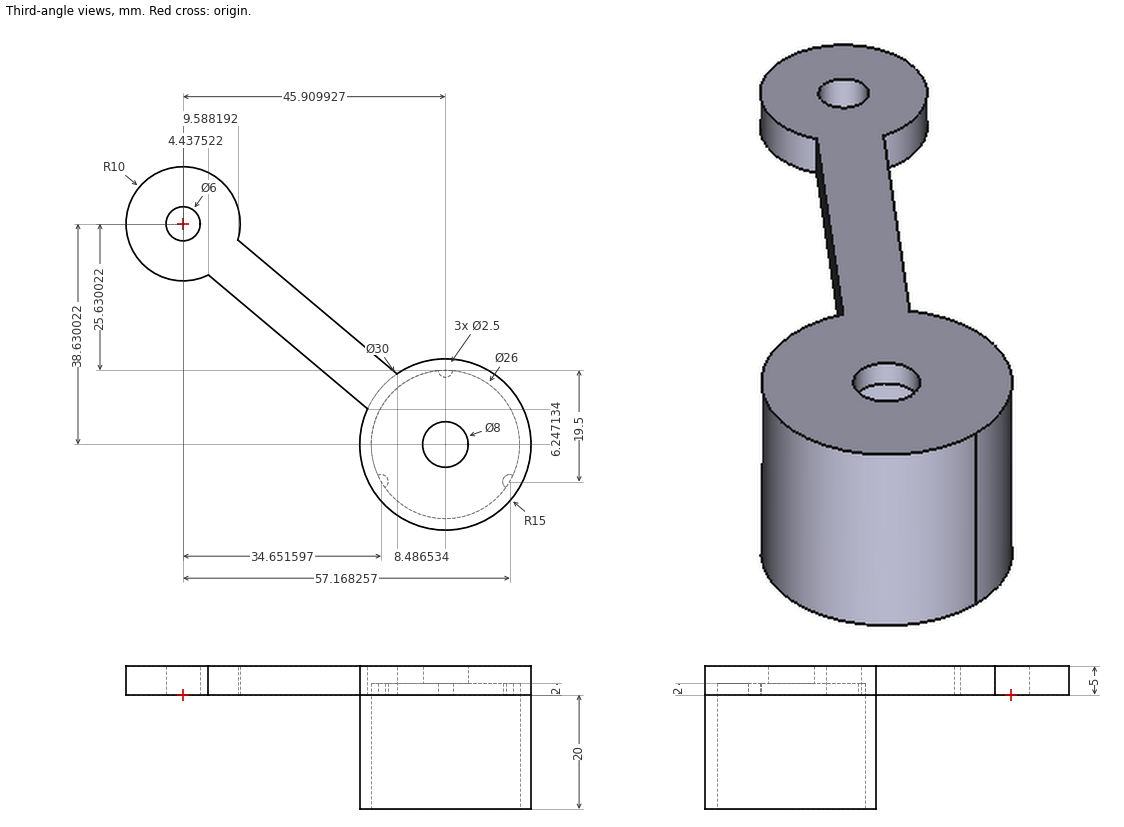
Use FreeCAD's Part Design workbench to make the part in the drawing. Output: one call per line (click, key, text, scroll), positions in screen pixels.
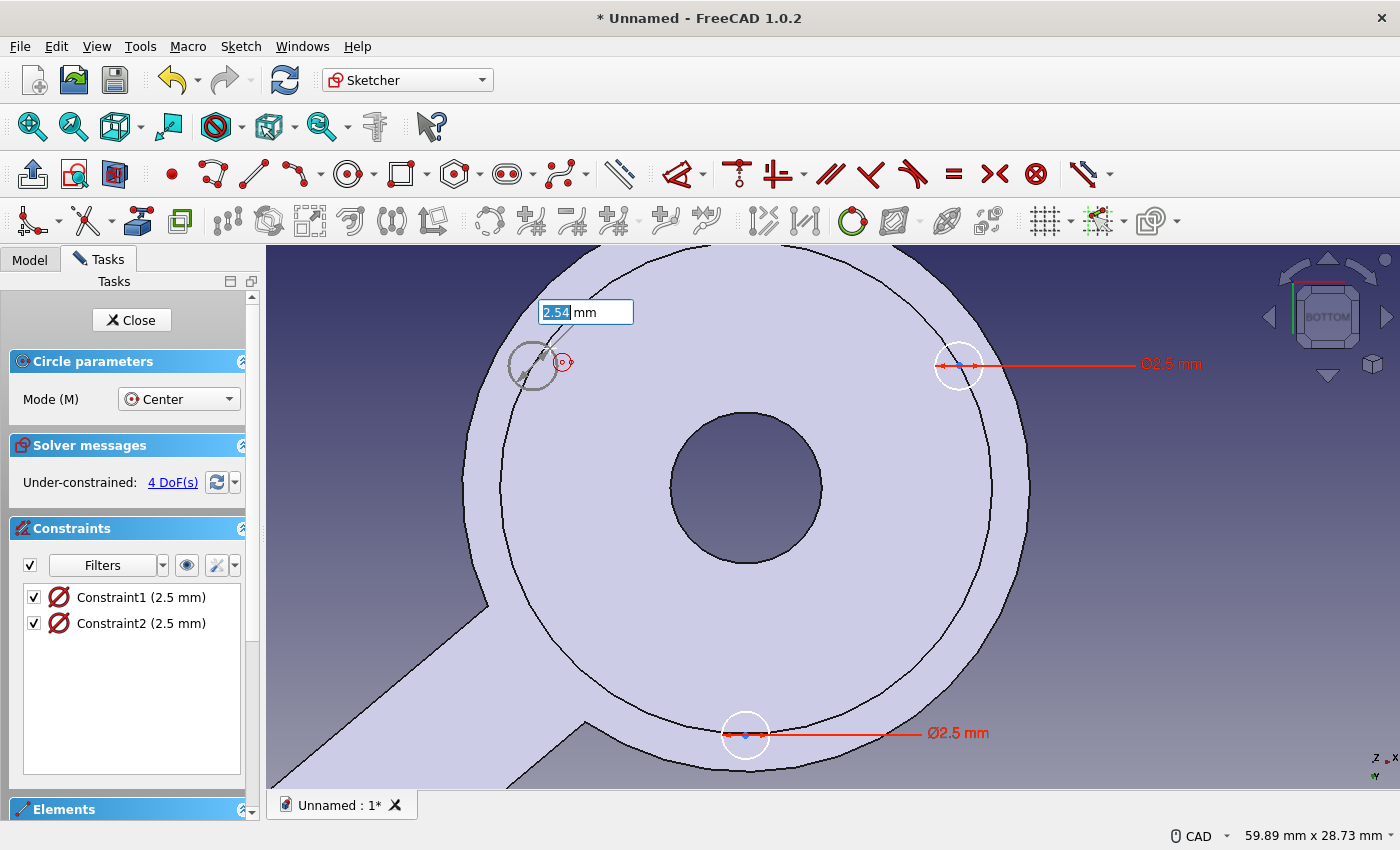
text(2.5)
key(Return)
key(Escape)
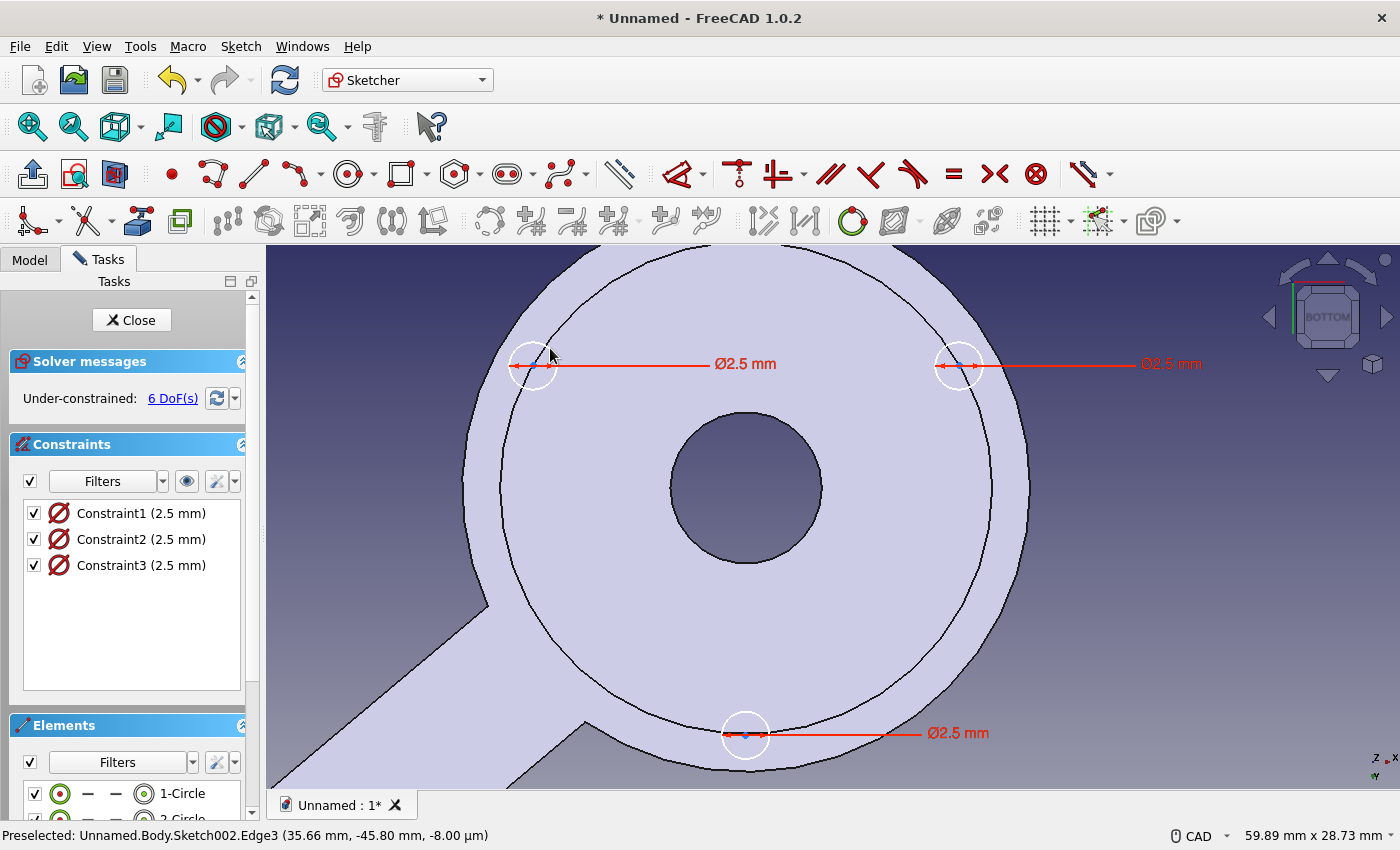
click(959, 366)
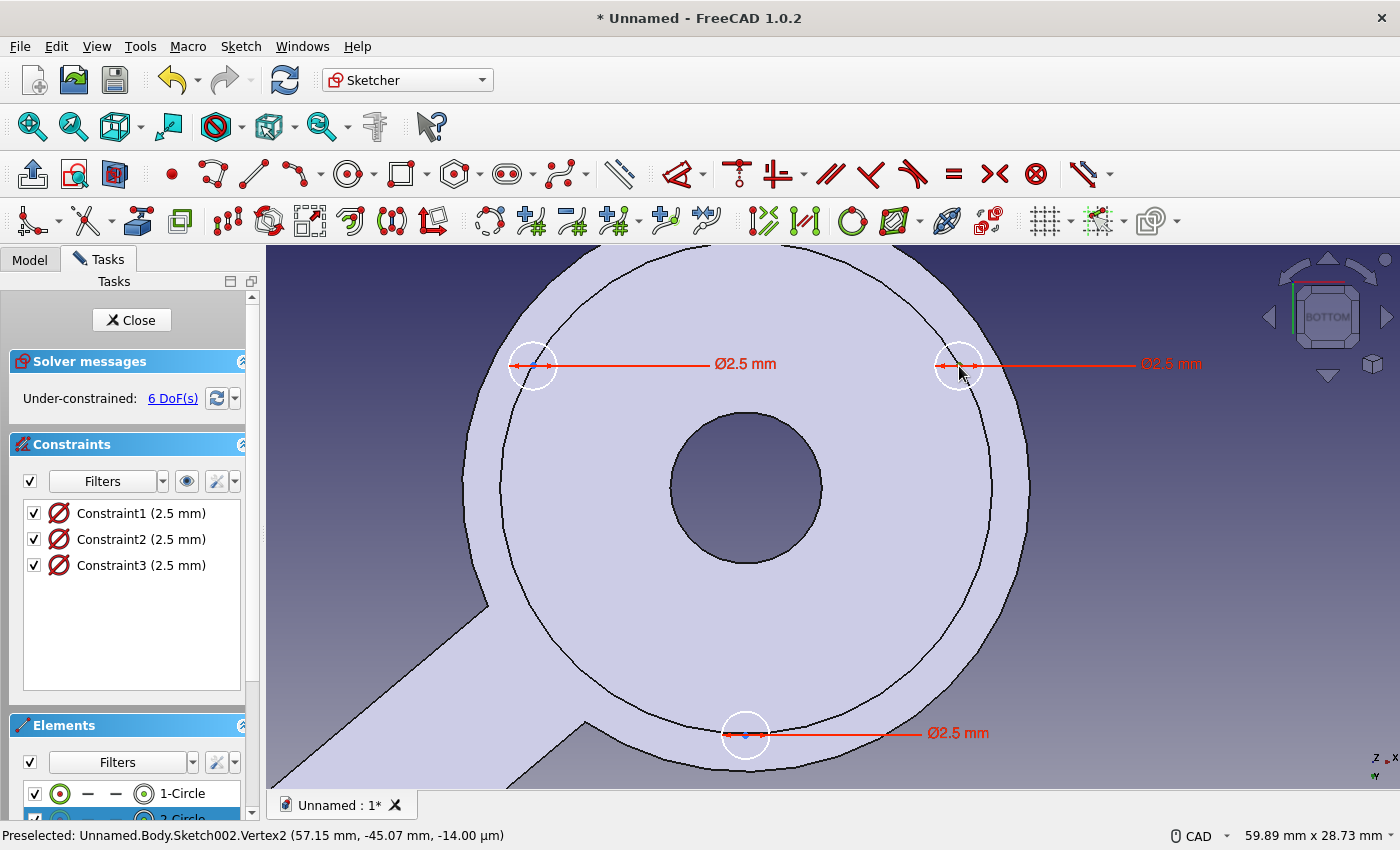
click(533, 366)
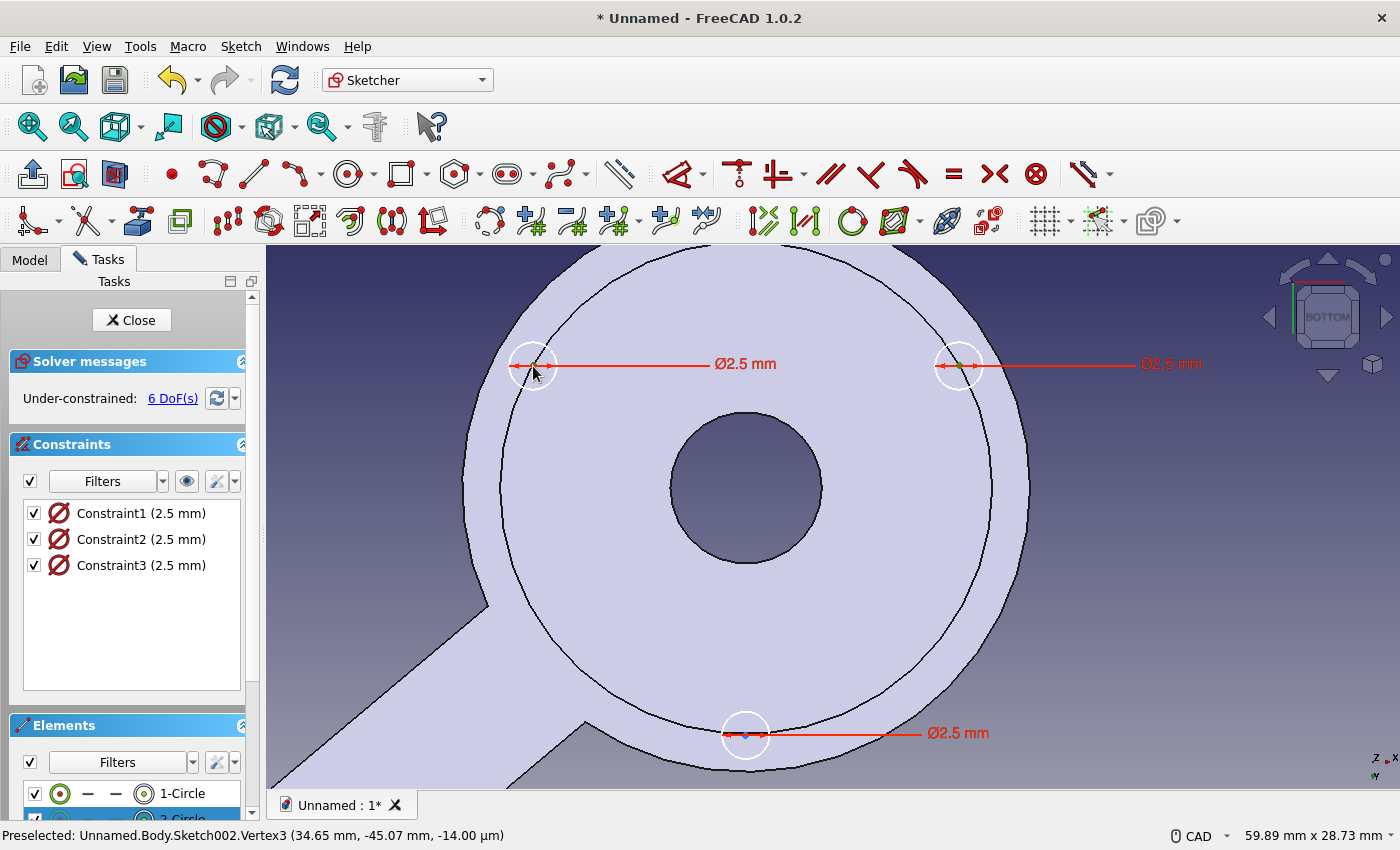
click(804, 174)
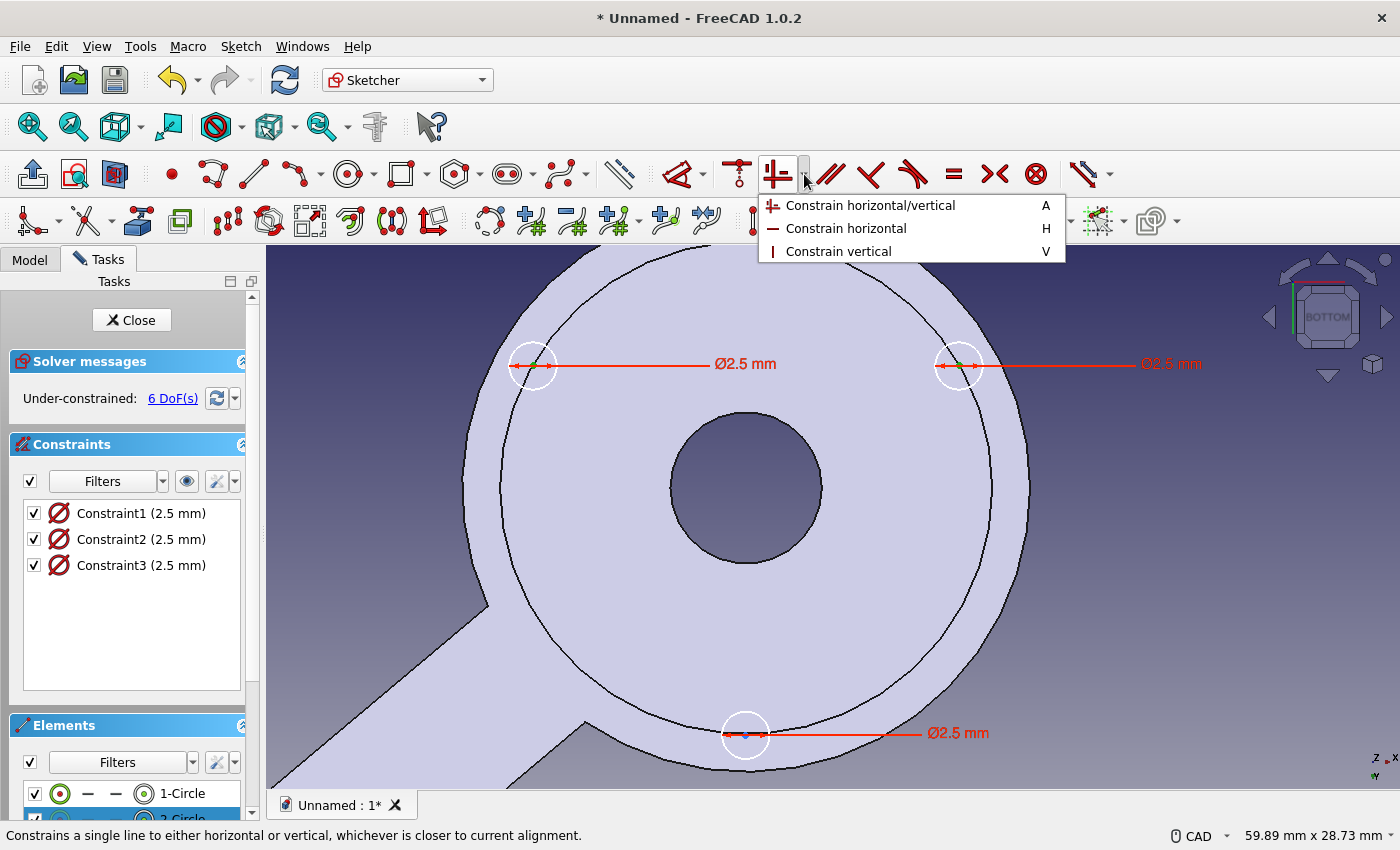
click(912, 228)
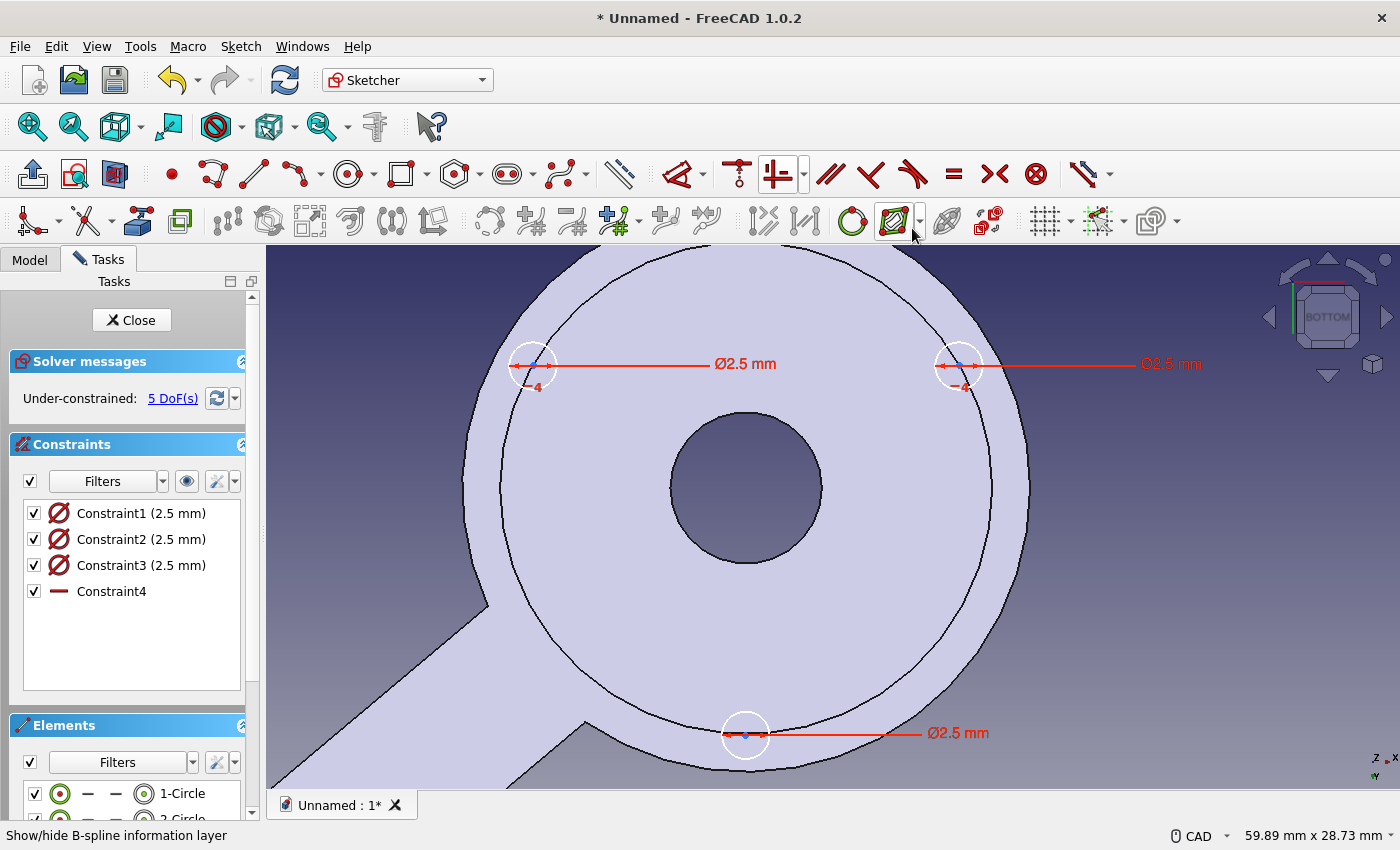
click(676, 174)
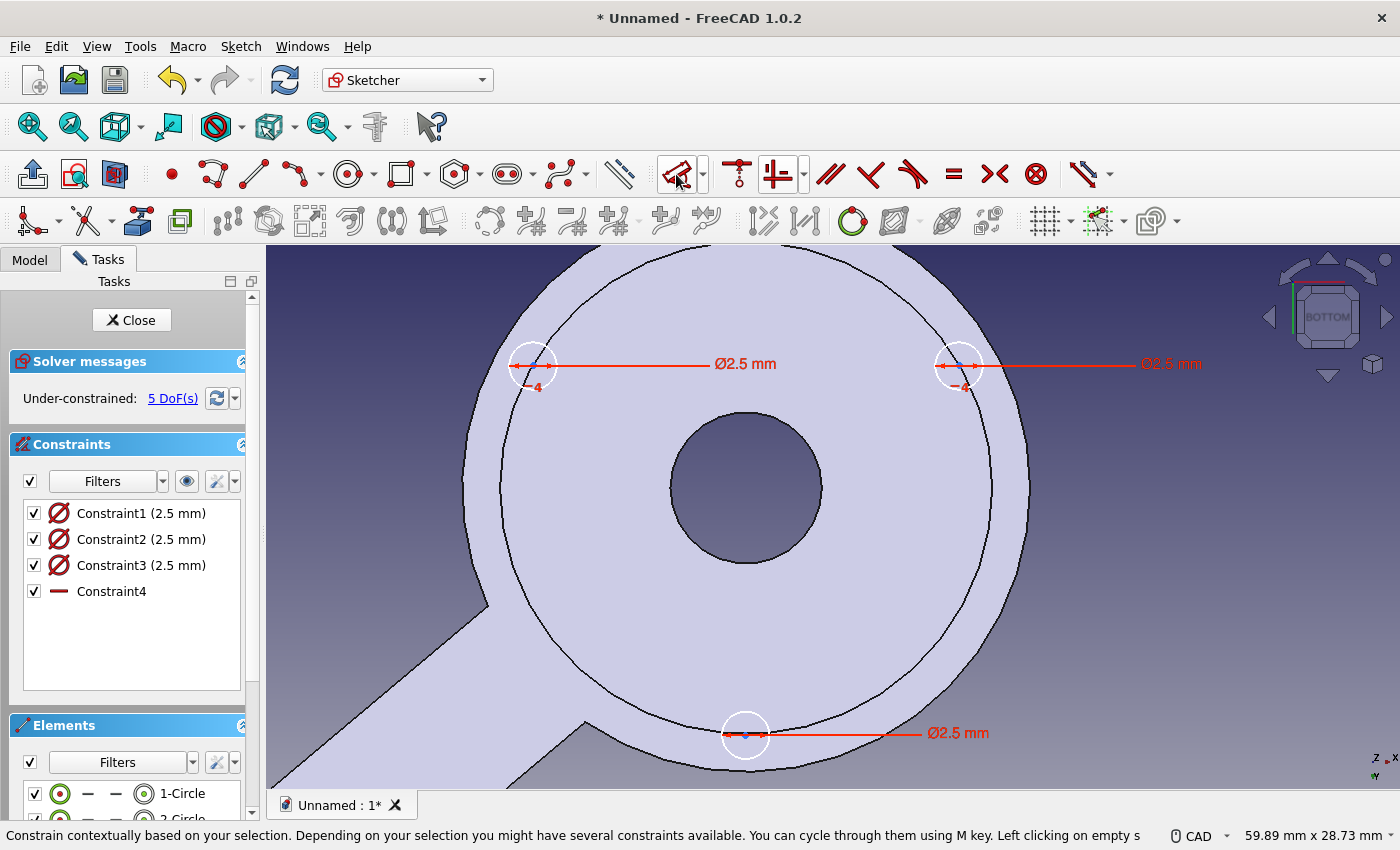
click(746, 735)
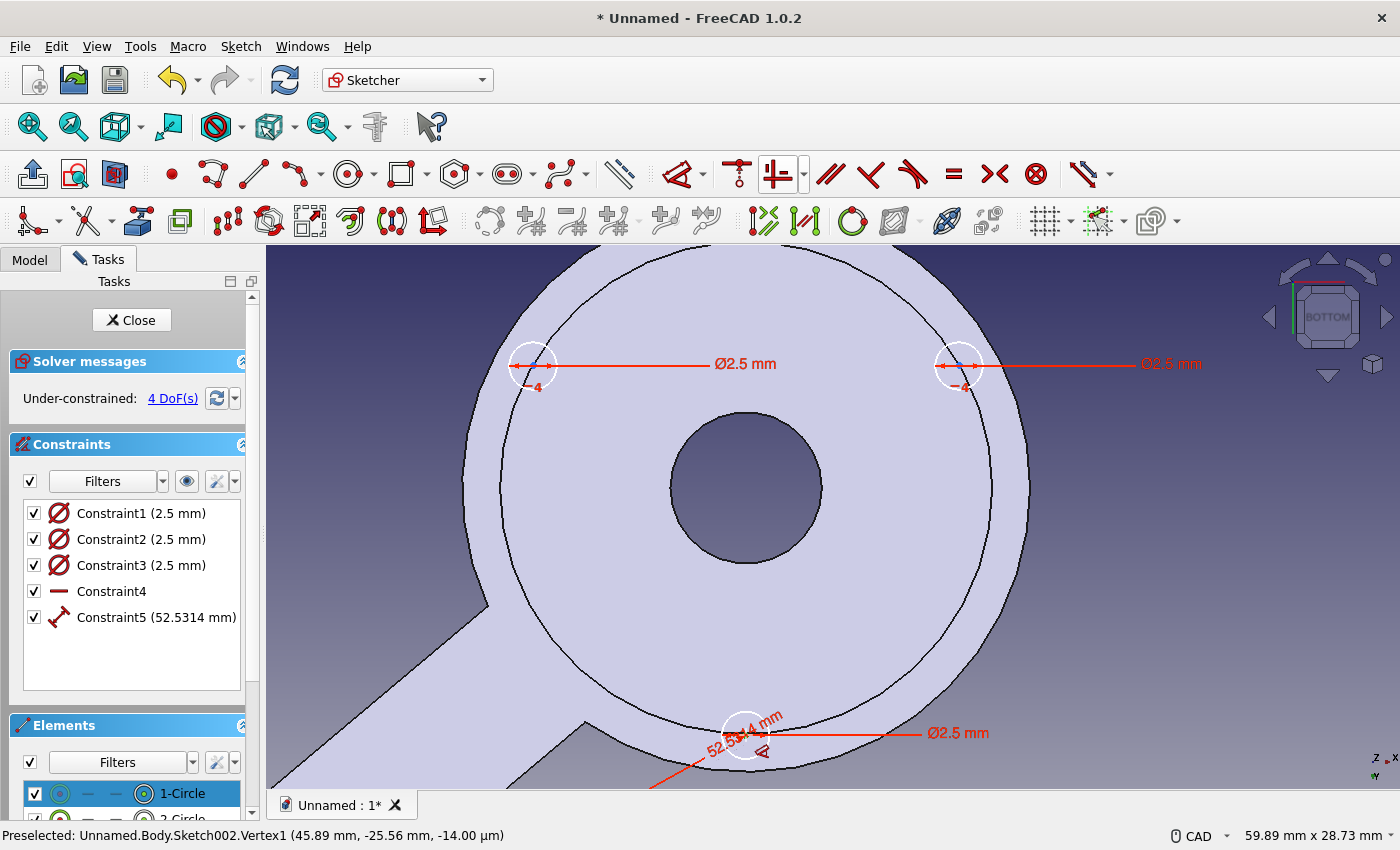
click(959, 366)
click(993, 551)